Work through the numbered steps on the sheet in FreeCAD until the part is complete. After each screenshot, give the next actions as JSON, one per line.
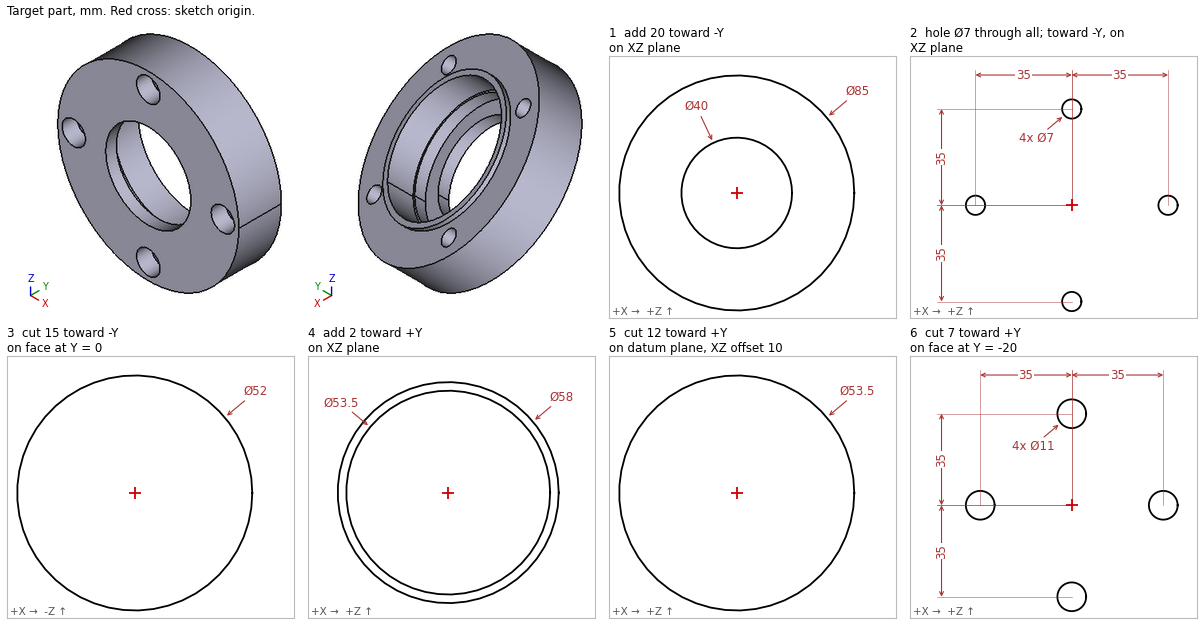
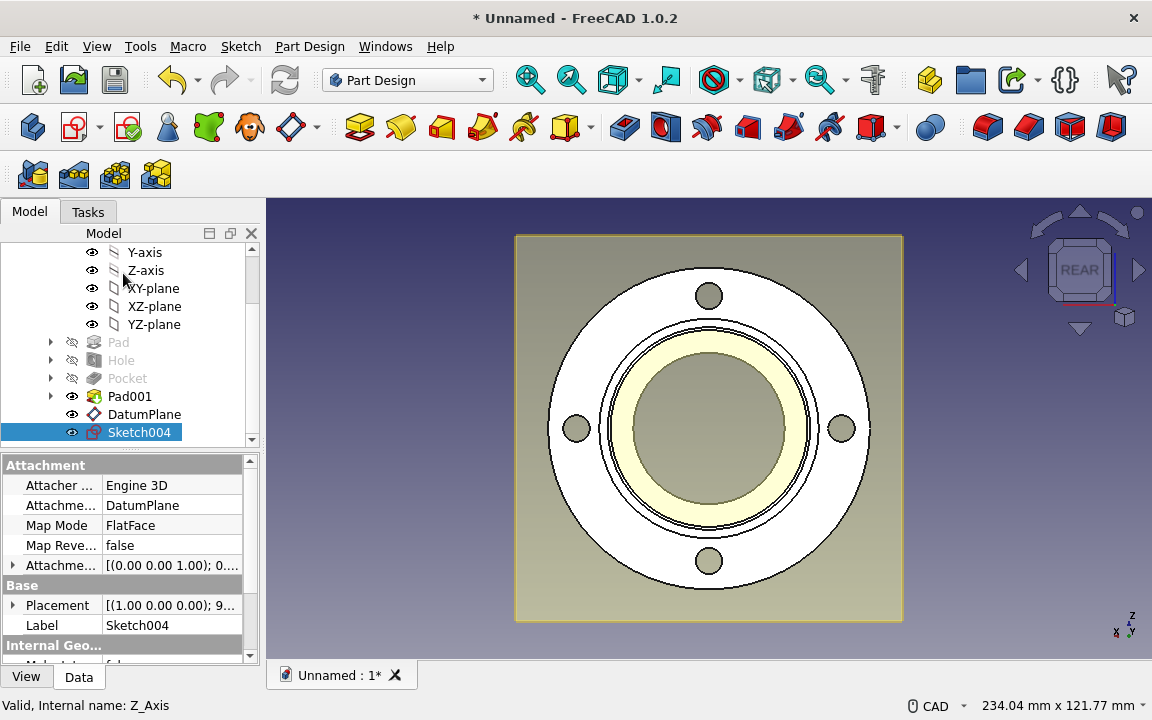
{"action": "left_click", "coordinate": [625, 128]}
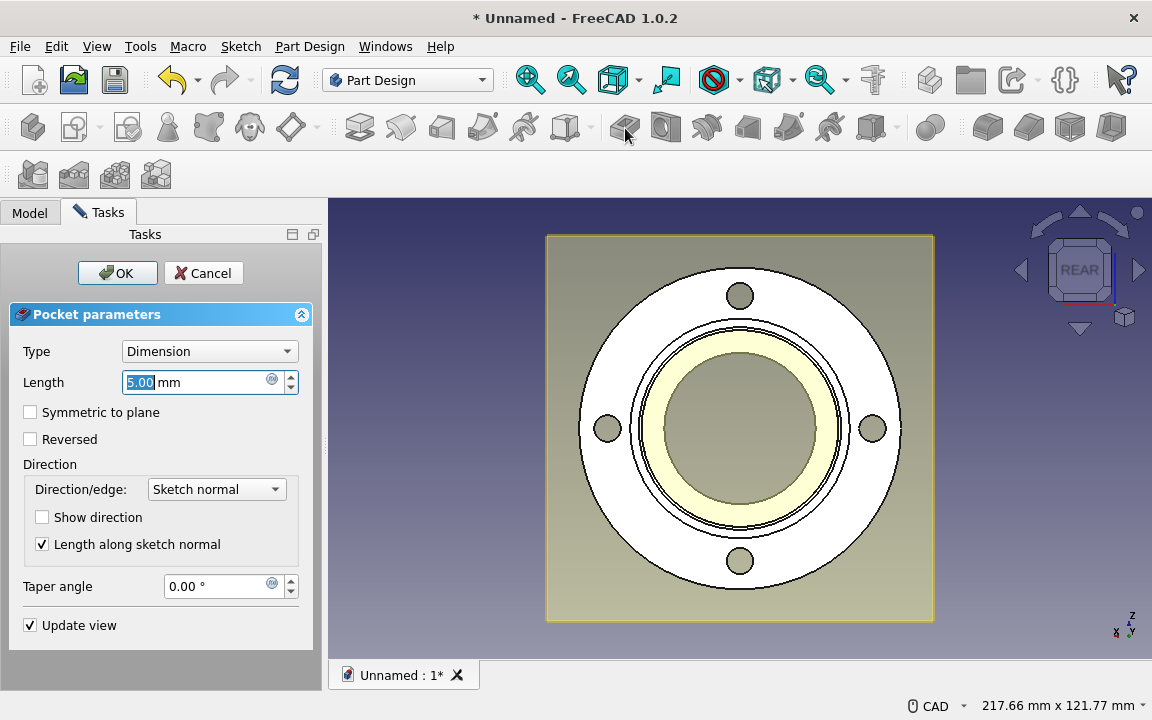
{"action": "type", "text": "12"}
{"action": "key", "text": "Tab"}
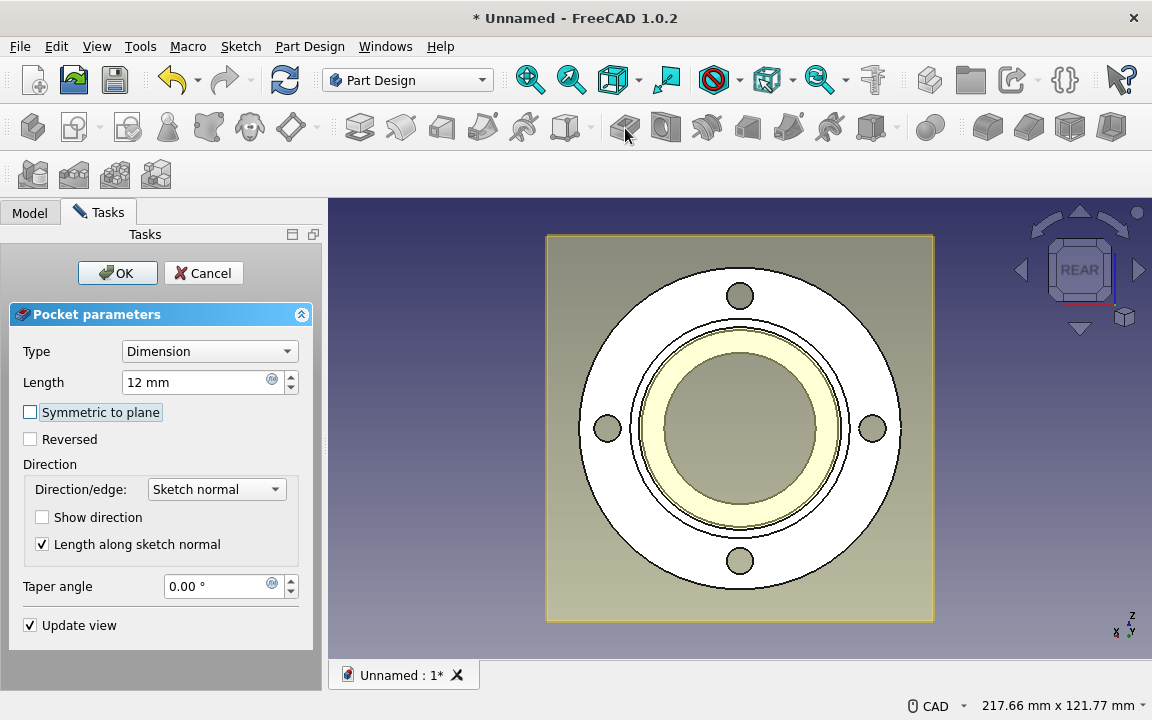
{"action": "left_click", "coordinate": [118, 273]}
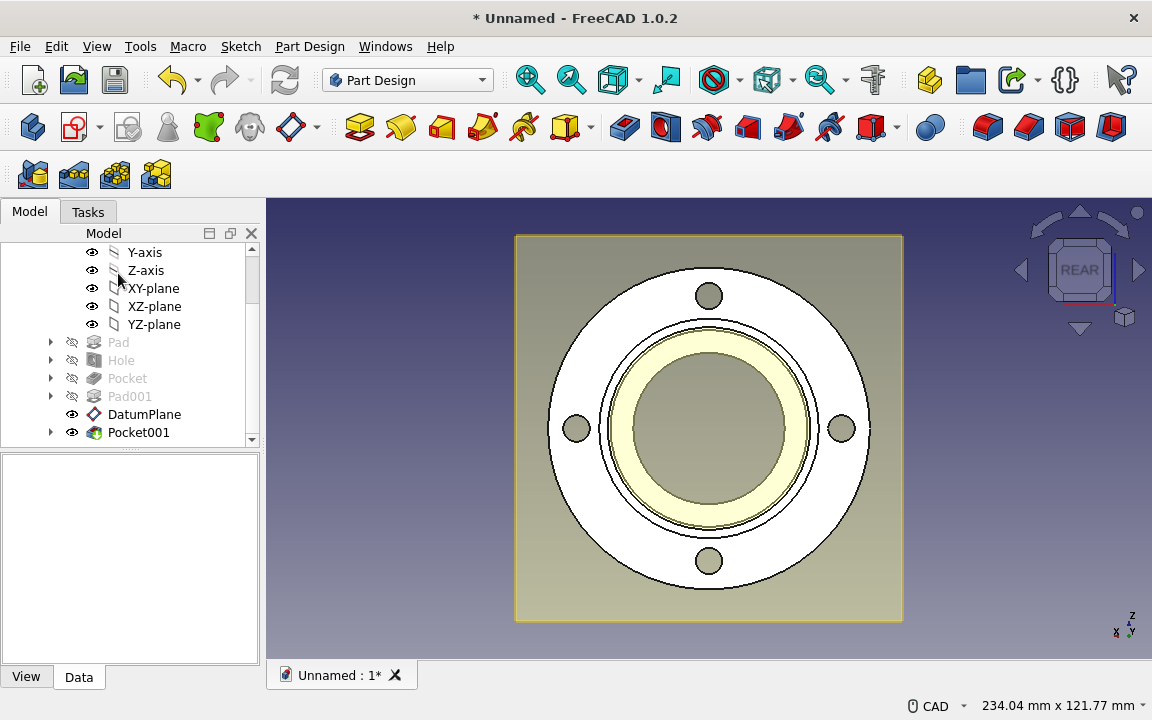
{"action": "left_click", "coordinate": [117, 414]}
{"action": "key", "text": "space"}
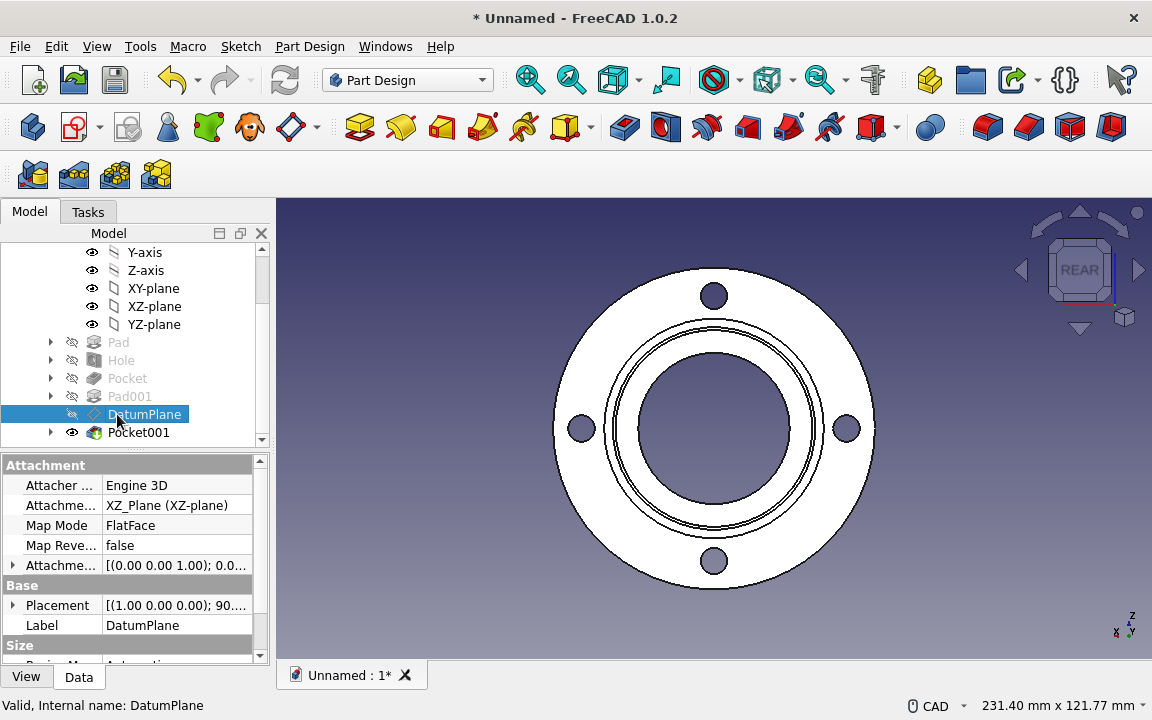
{"action": "key", "text": "0"}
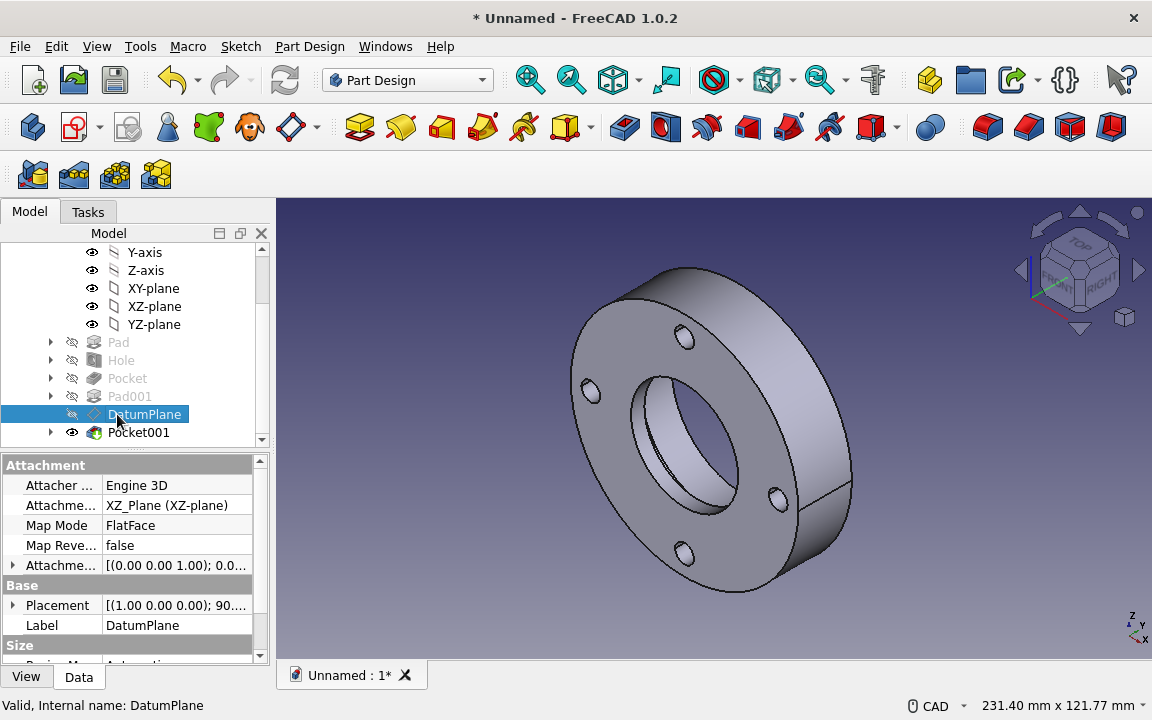
{"action": "left_click", "coordinate": [750, 557]}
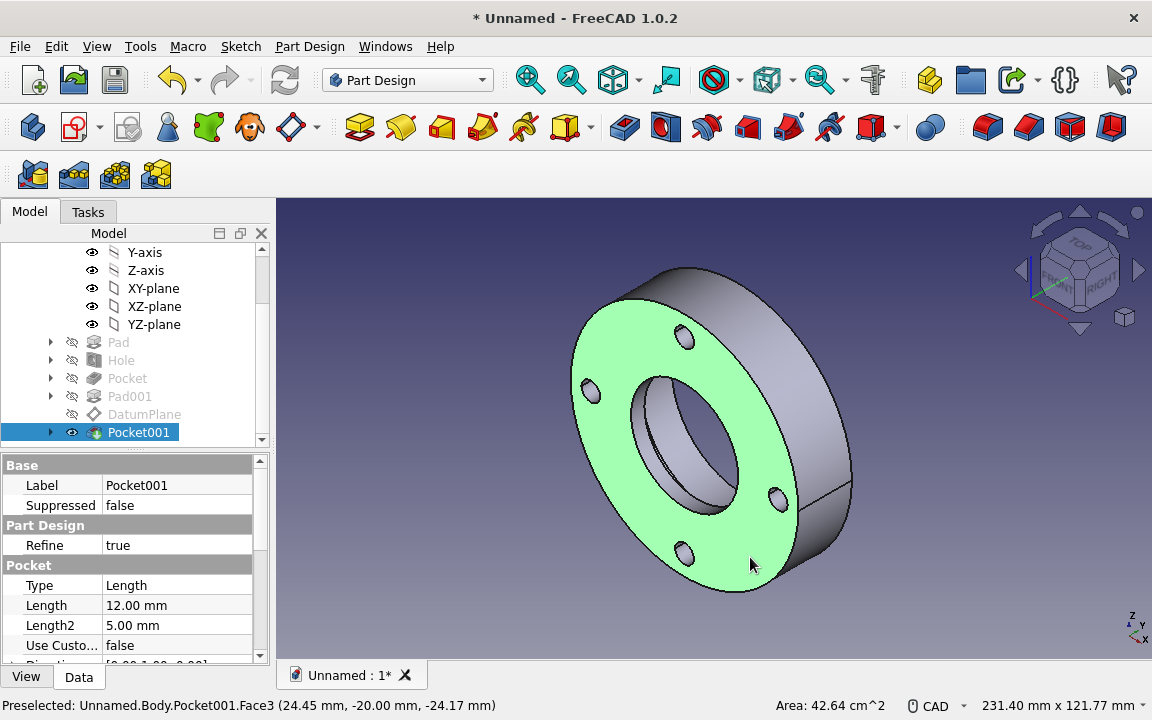
{"action": "left_click", "coordinate": [74, 128]}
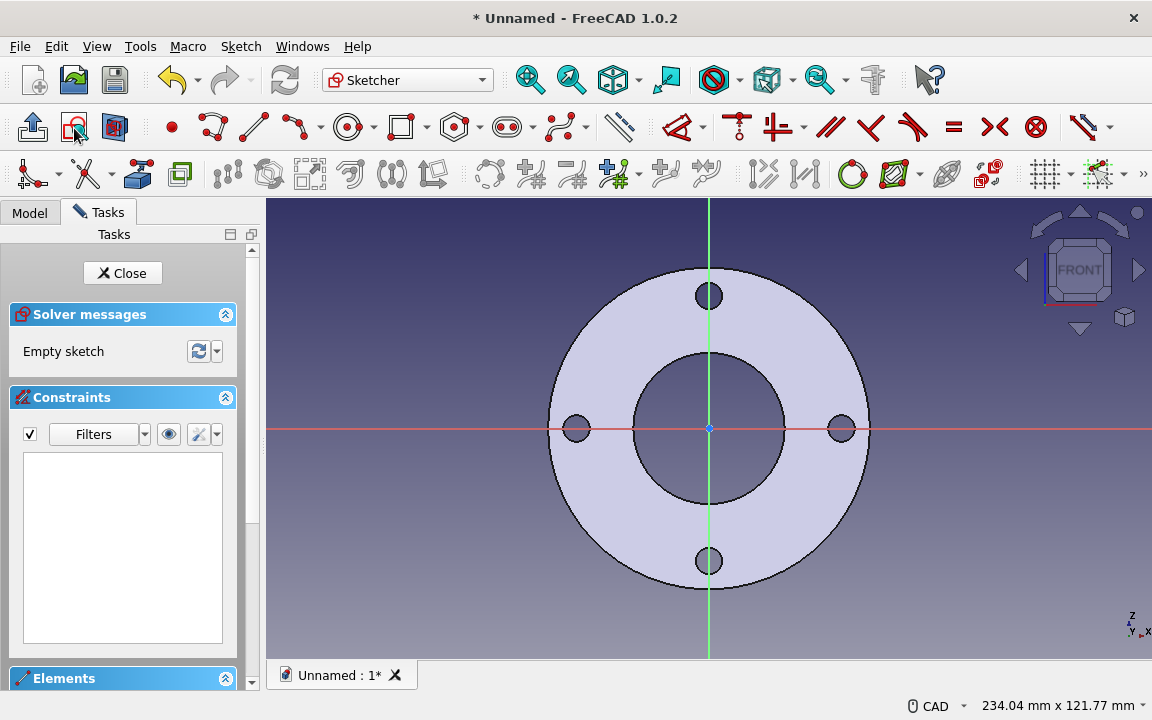
{"action": "key", "text": "g c"}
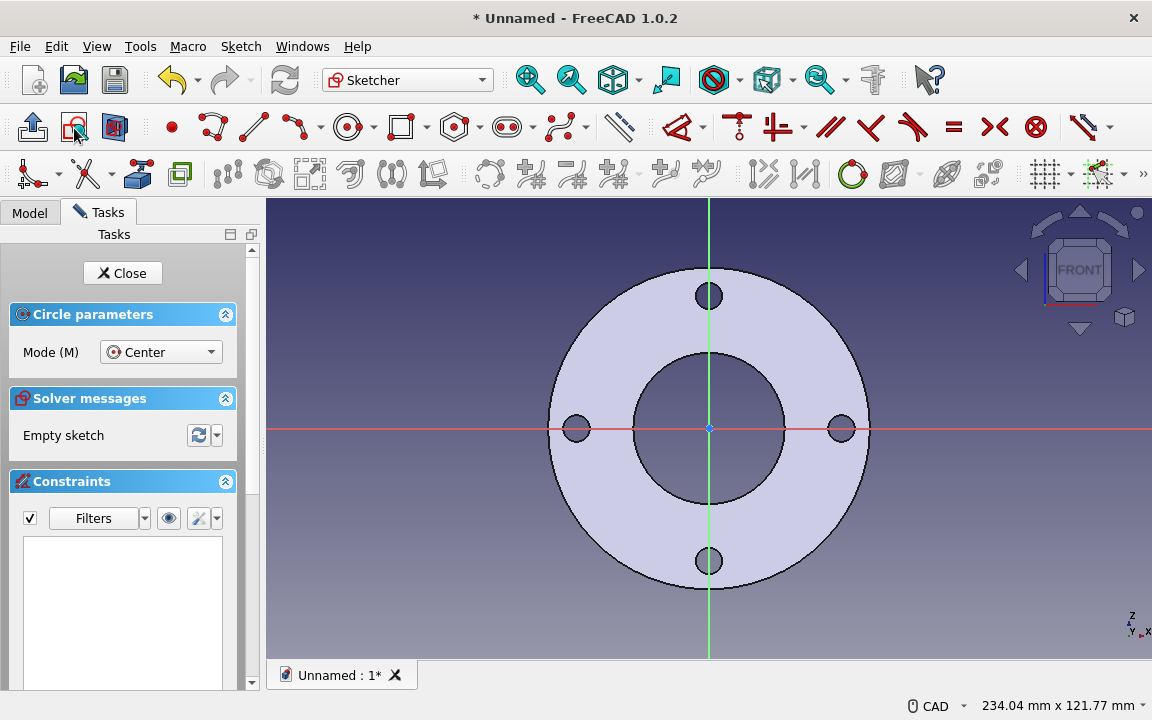
{"action": "left_click", "coordinate": [709, 296]}
{"action": "mouse_move", "coordinate": [724, 281]}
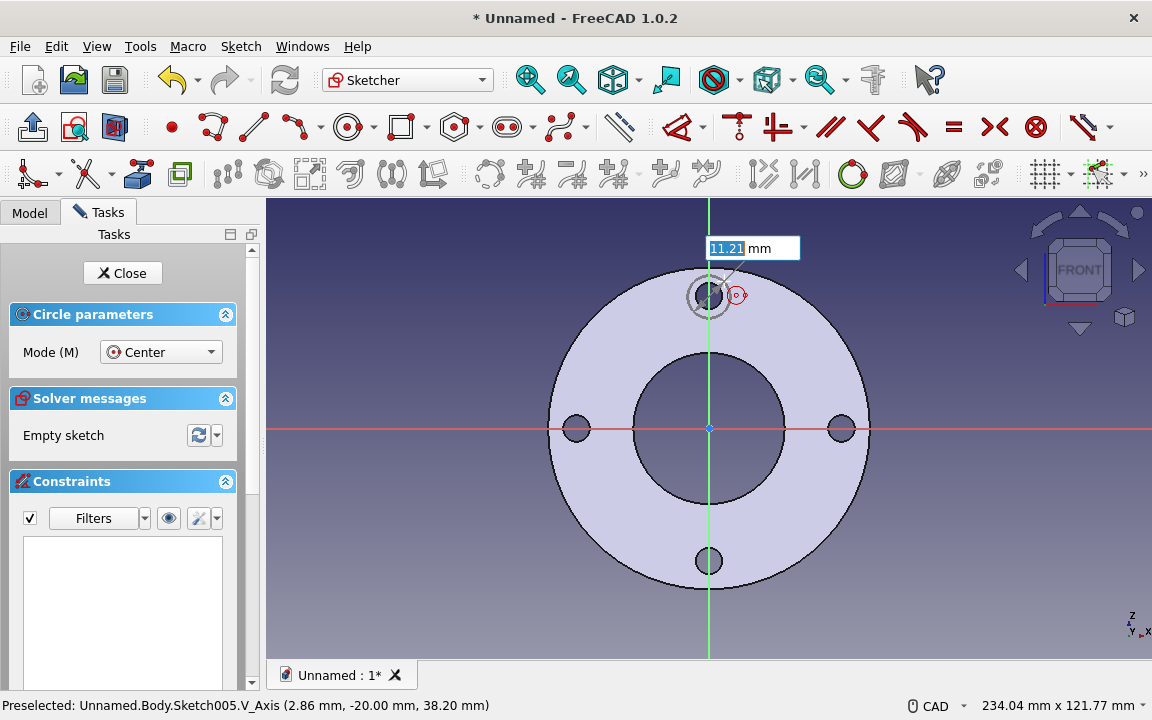
{"action": "type", "text": "11"}
{"action": "key", "text": "Return"}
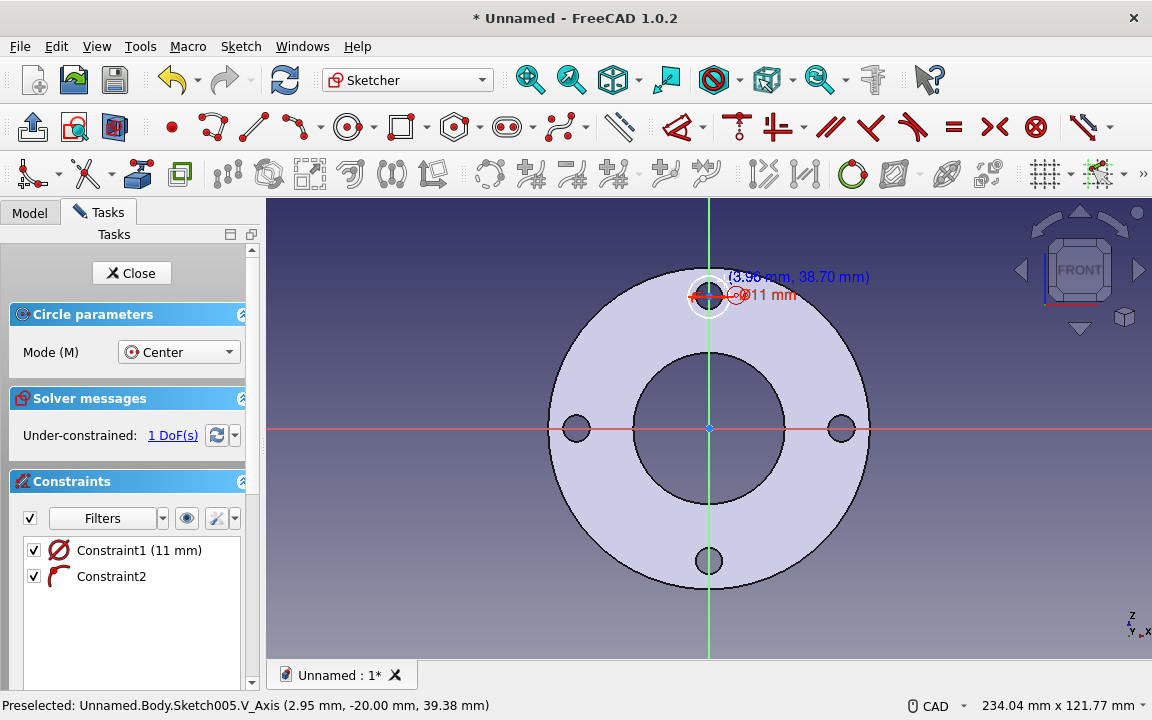
{"action": "left_click", "coordinate": [577, 428]}
{"action": "mouse_move", "coordinate": [591, 414]}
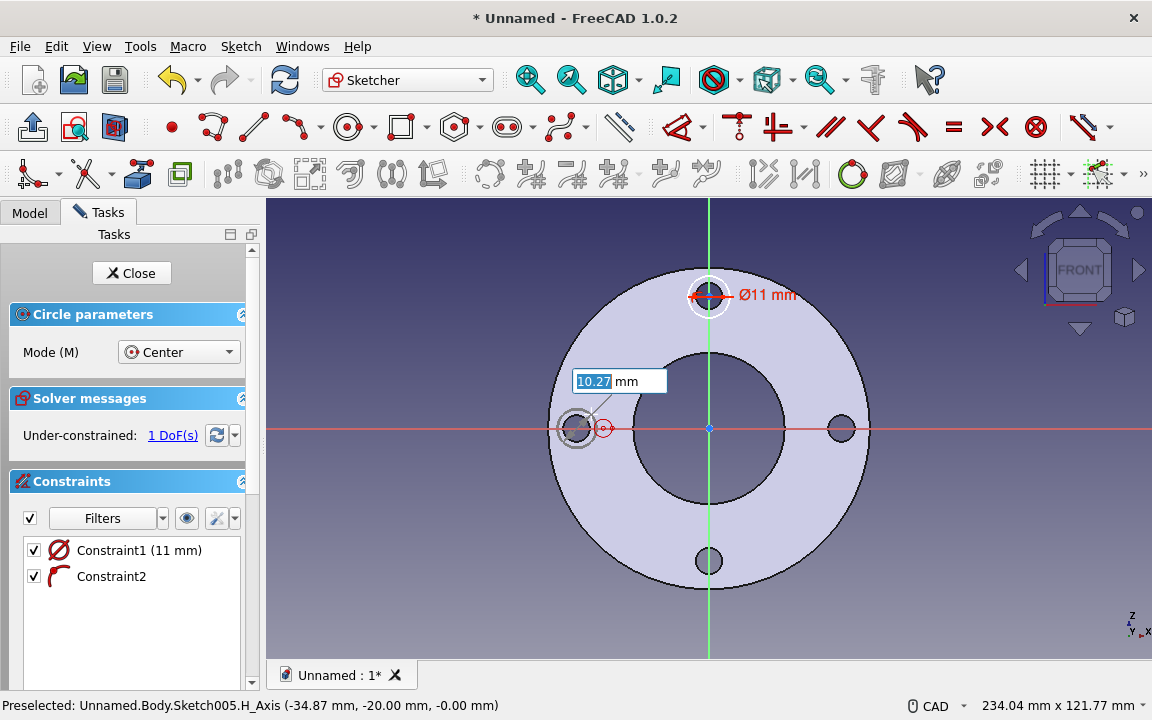
{"action": "type", "text": "11"}
{"action": "key", "text": "Return"}